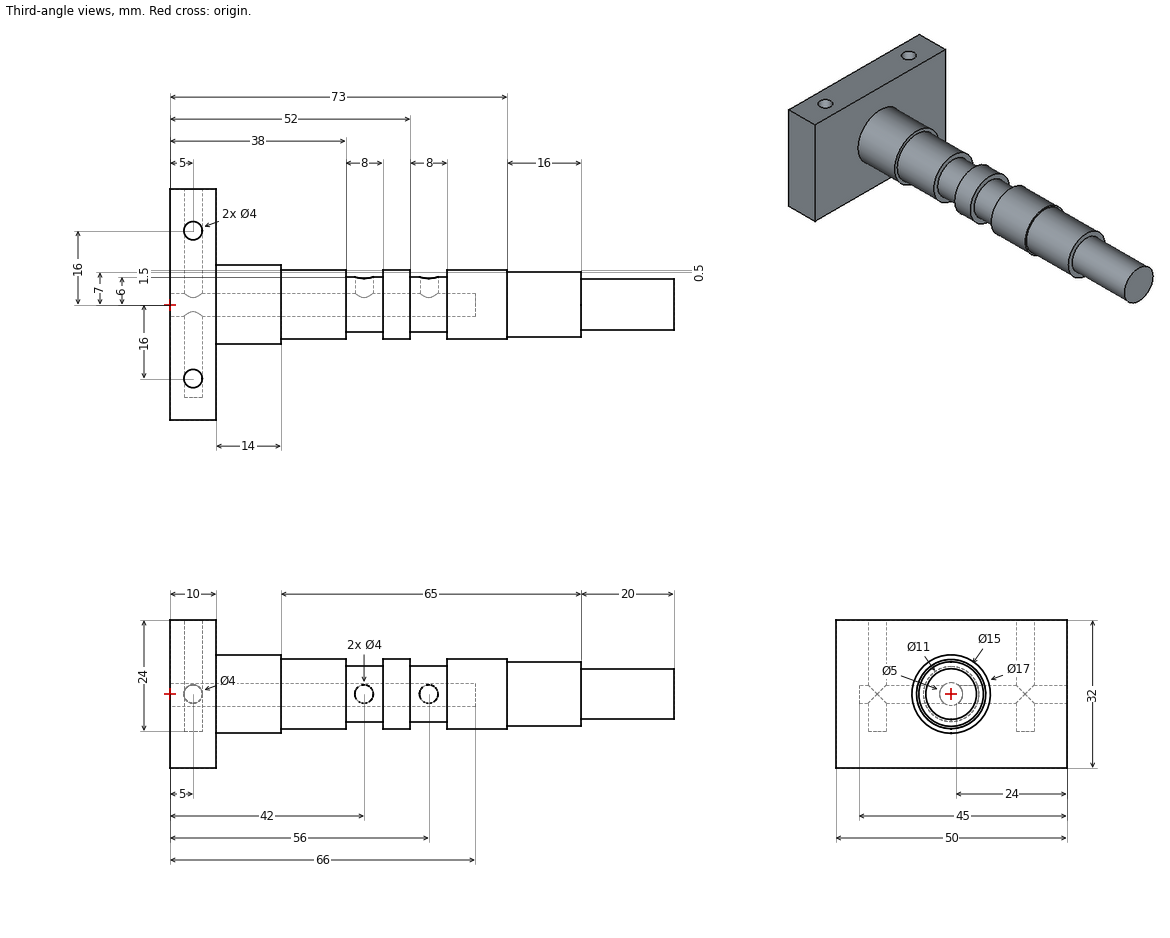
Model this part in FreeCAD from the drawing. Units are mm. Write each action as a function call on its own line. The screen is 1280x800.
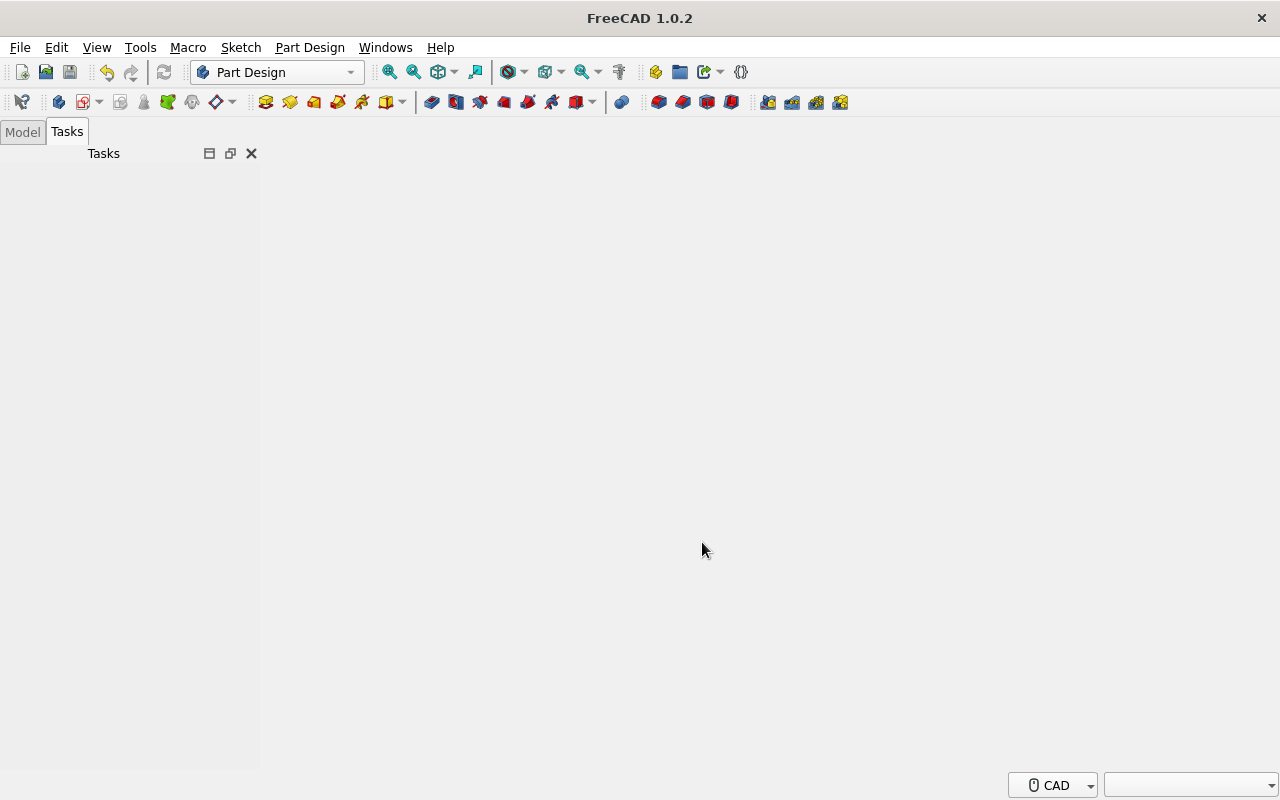
click(22, 72)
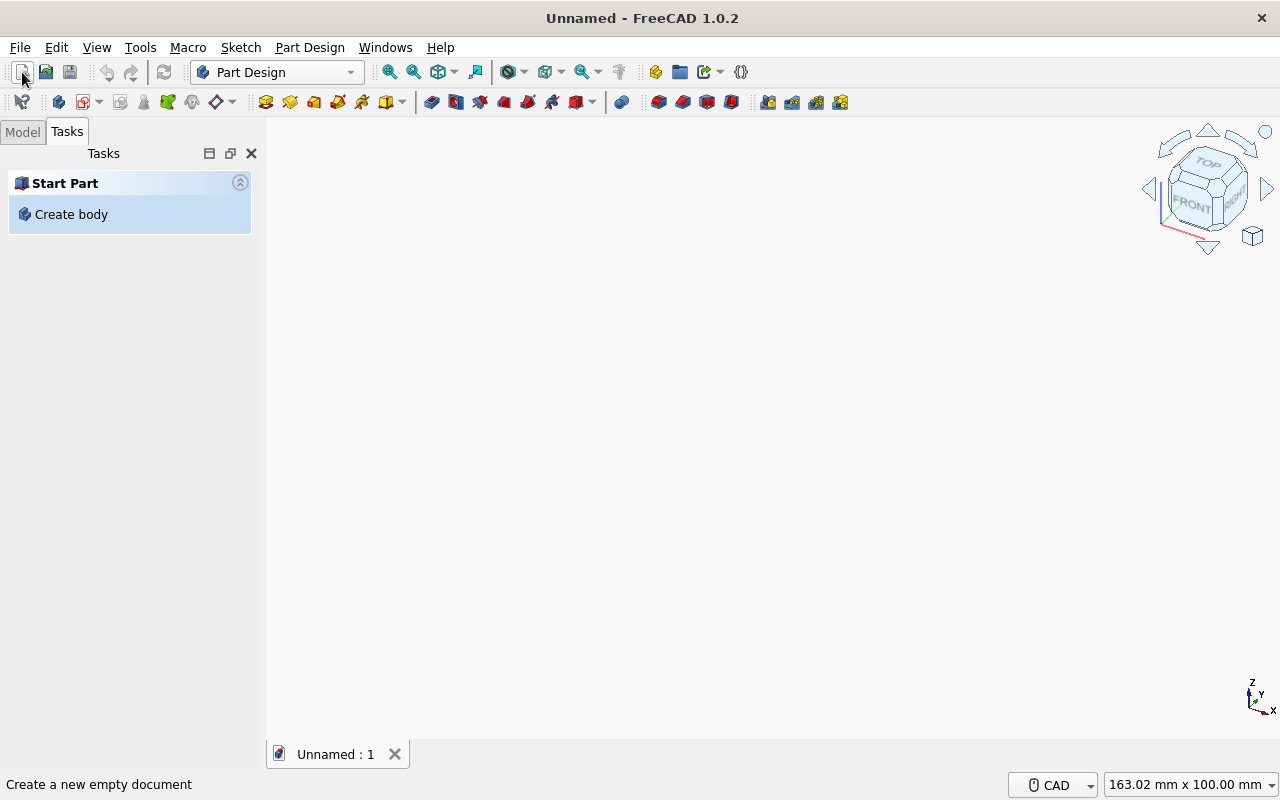
click(84, 102)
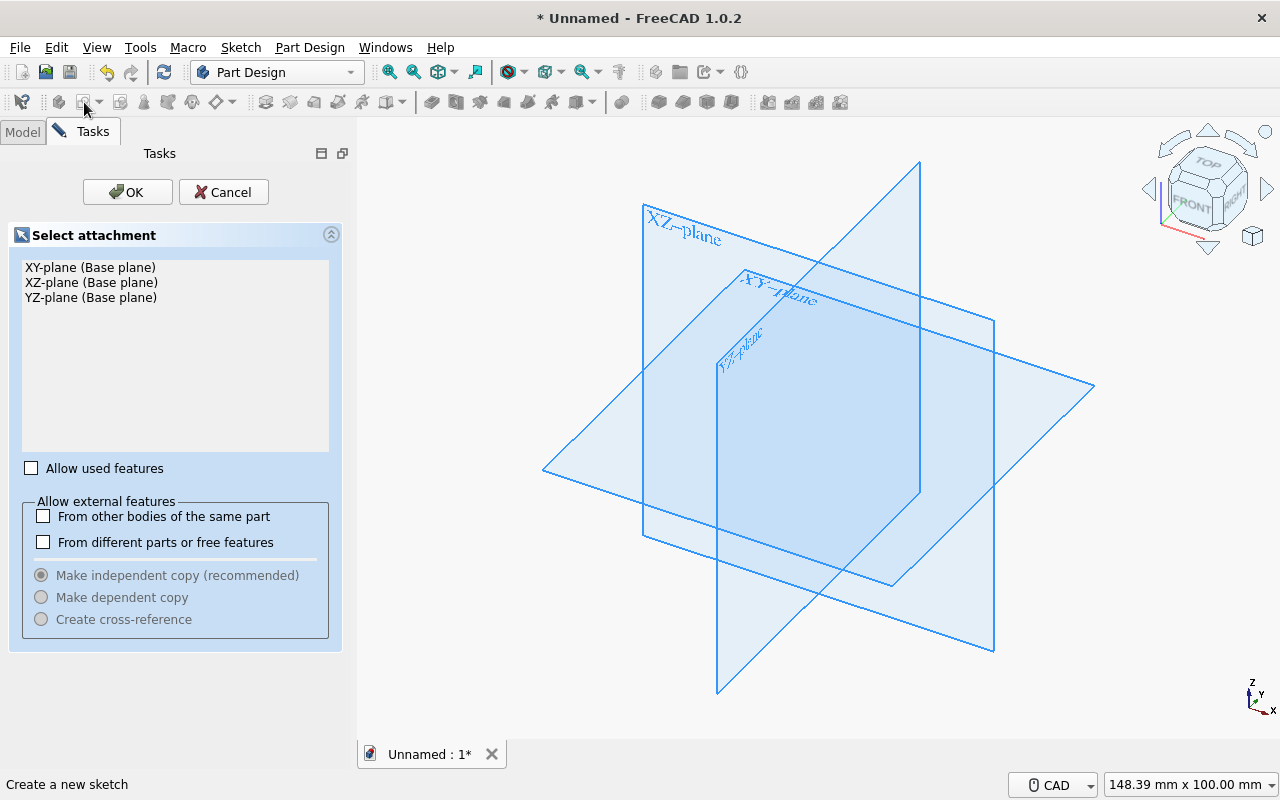
click(82, 298)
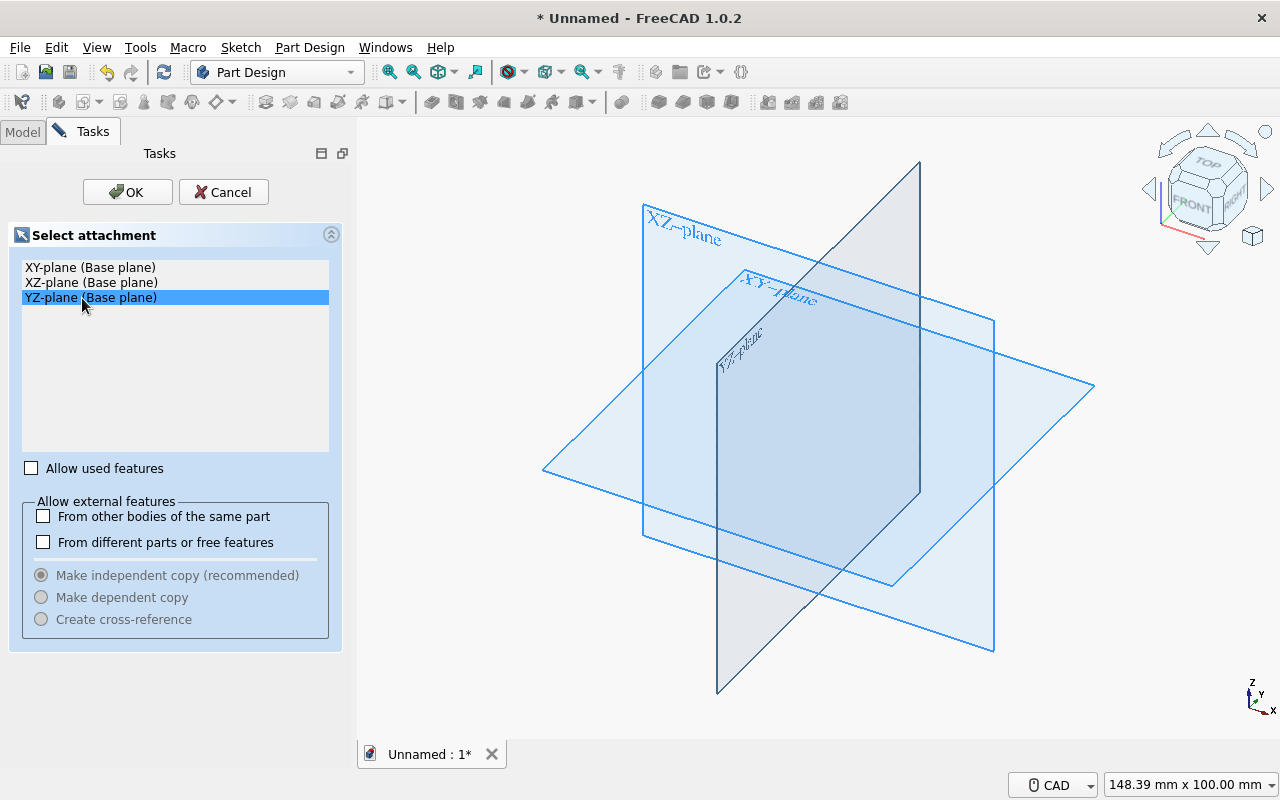
click(128, 192)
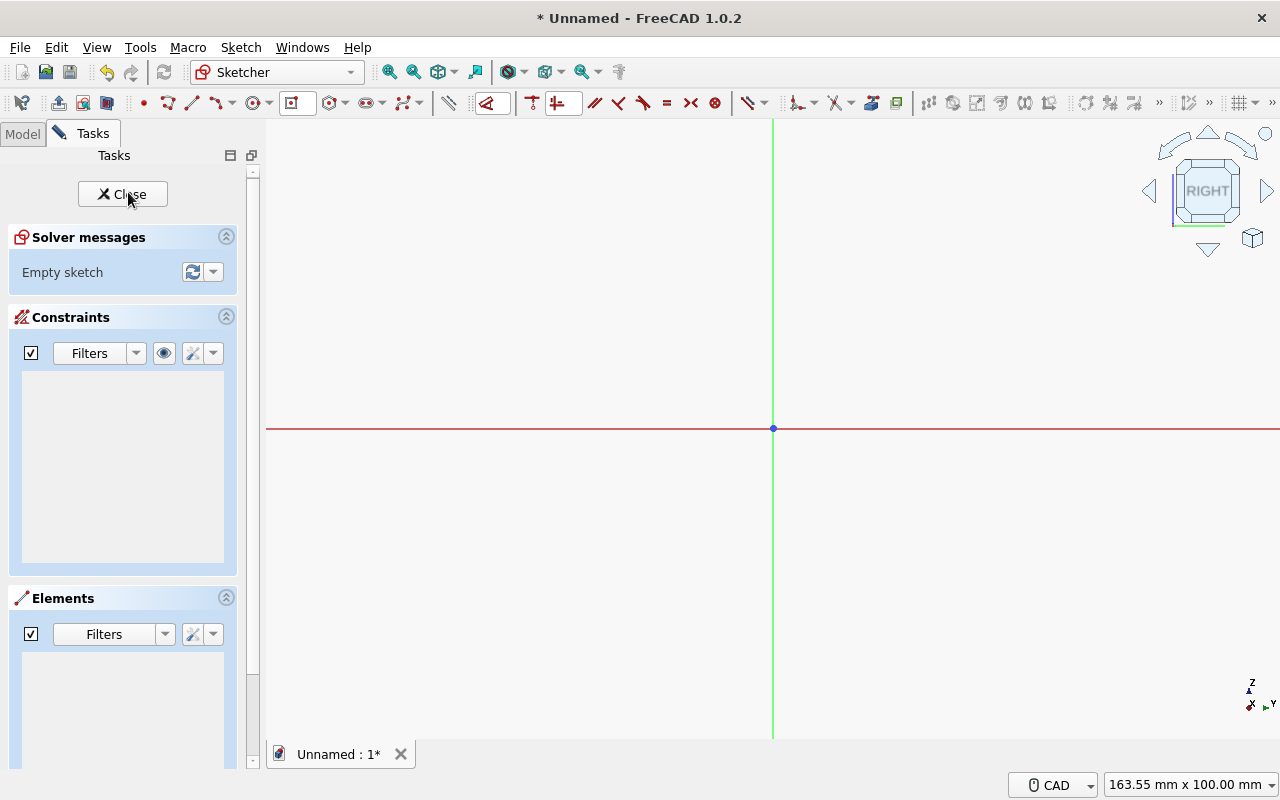
scroll(856, 429, up, 3)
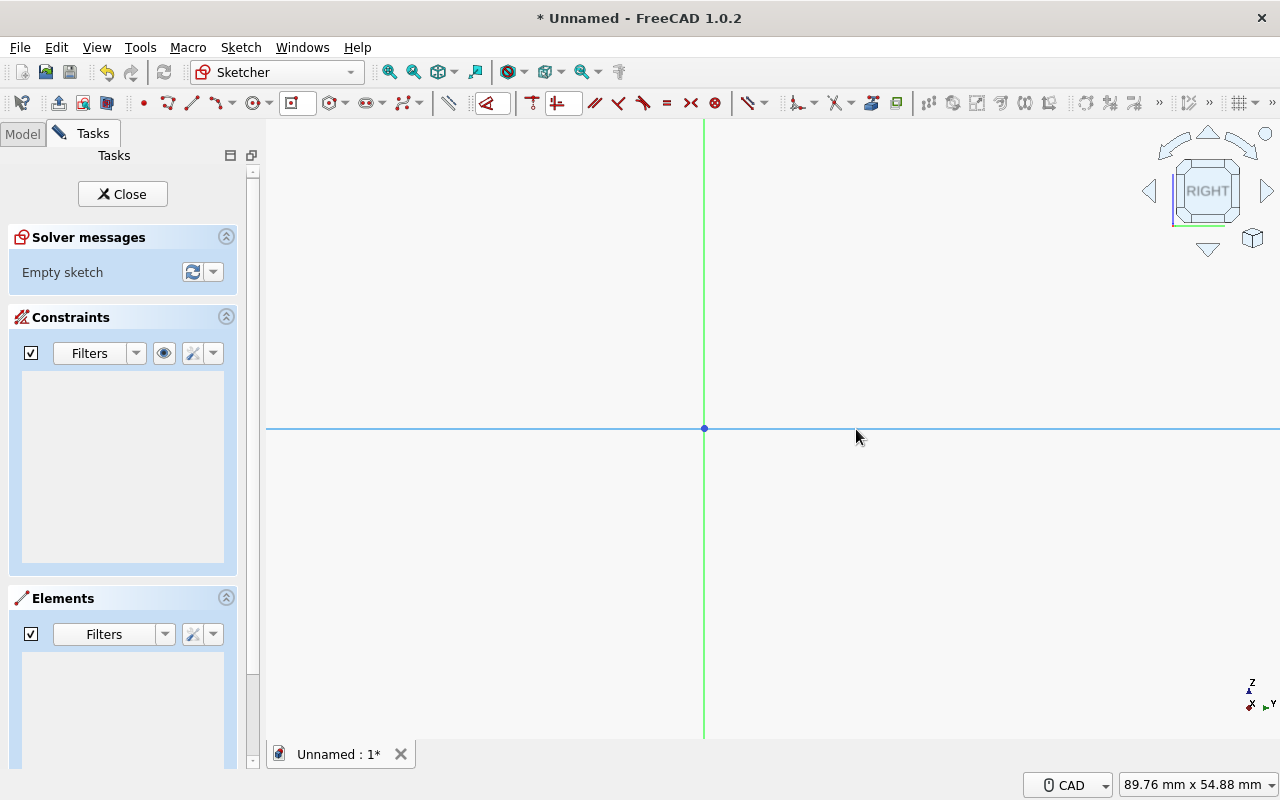
click(292, 104)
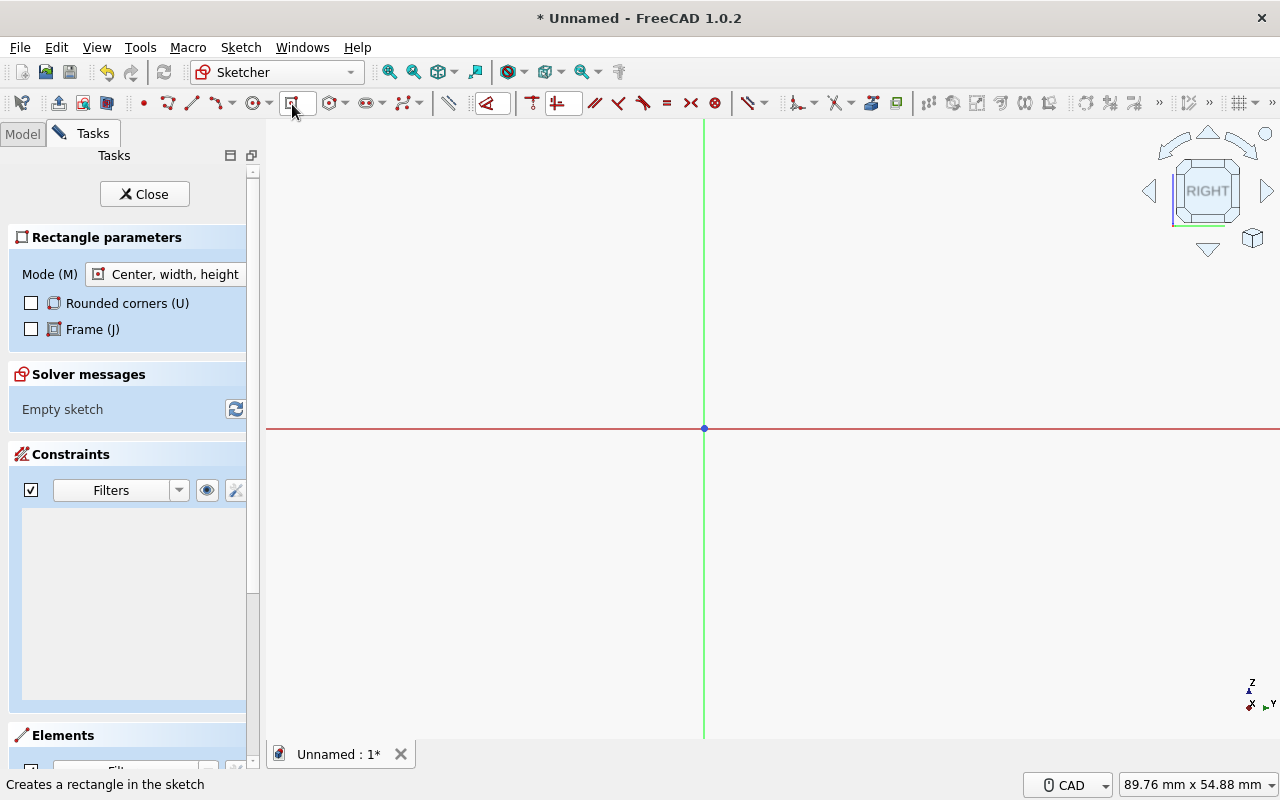
click(704, 429)
move(987, 248)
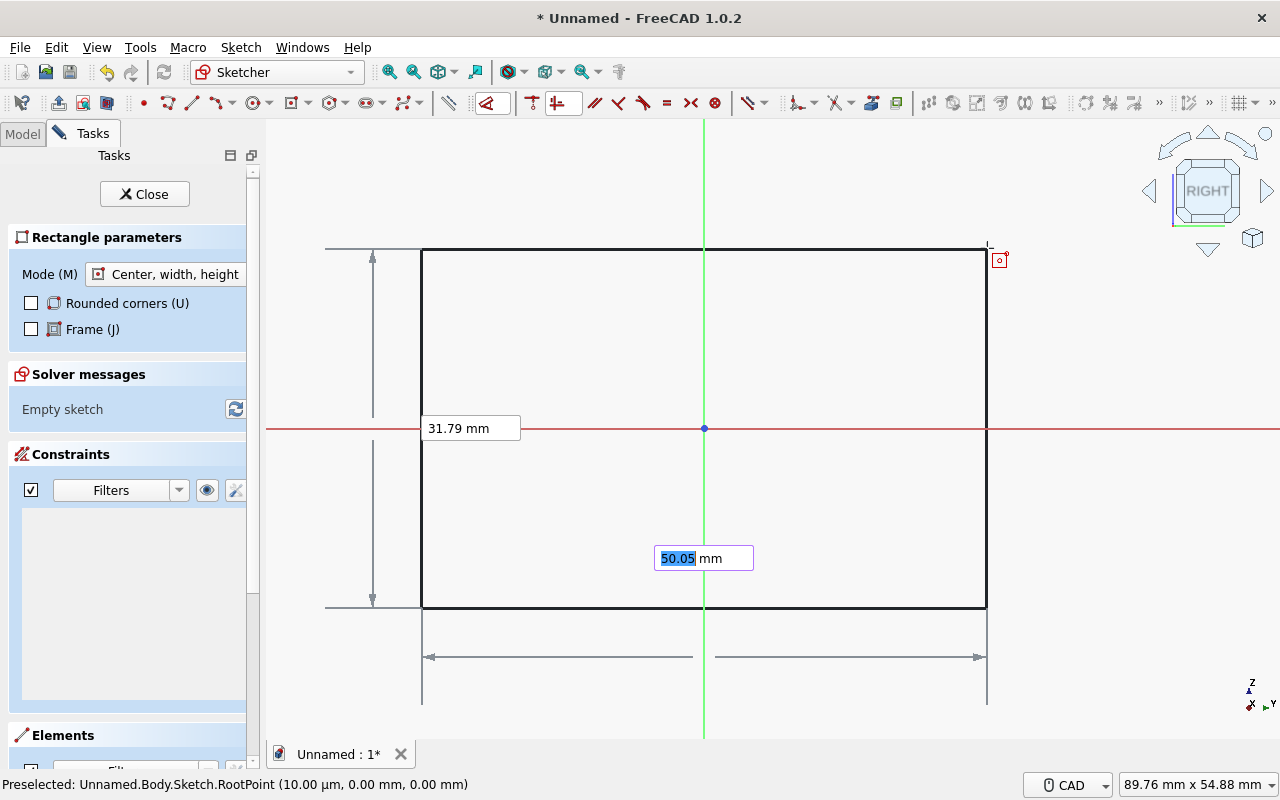
text(50)
key(Tab)
text(32)
key(Return)
key(Escape)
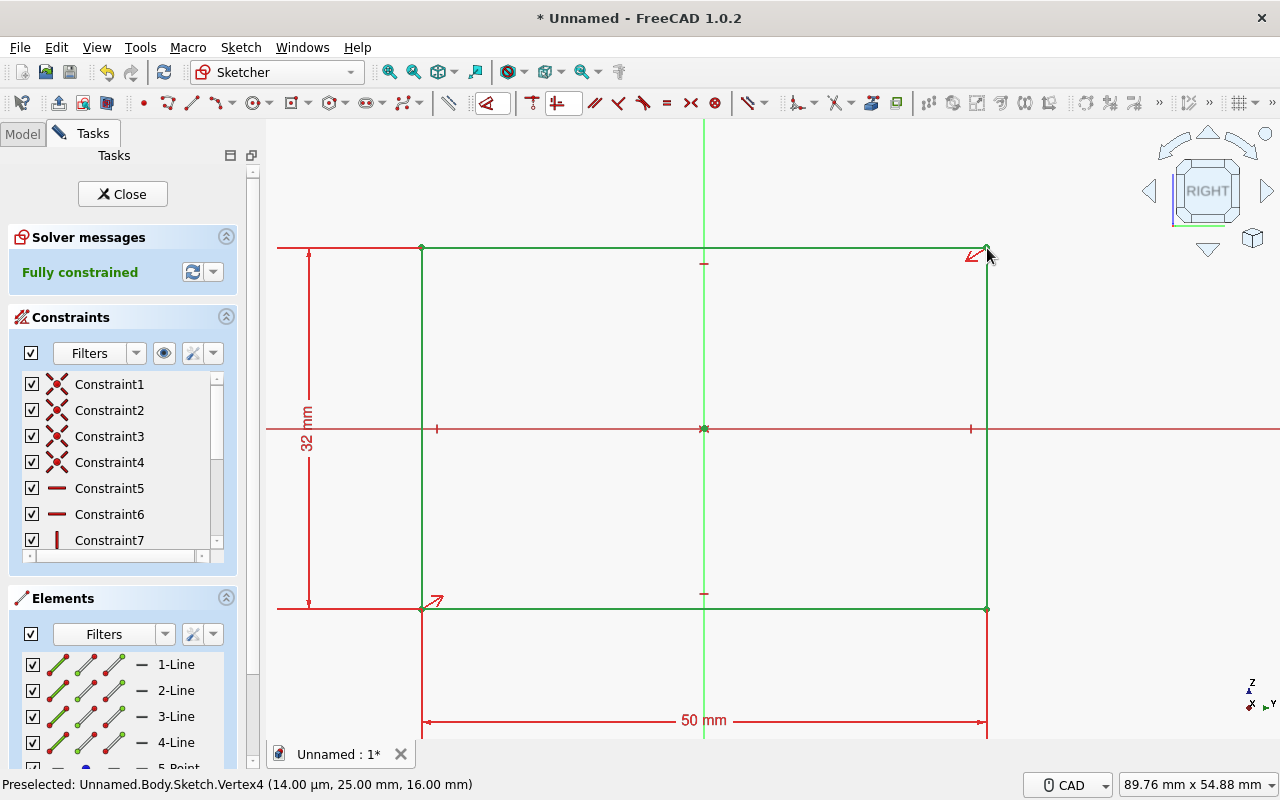
click(123, 194)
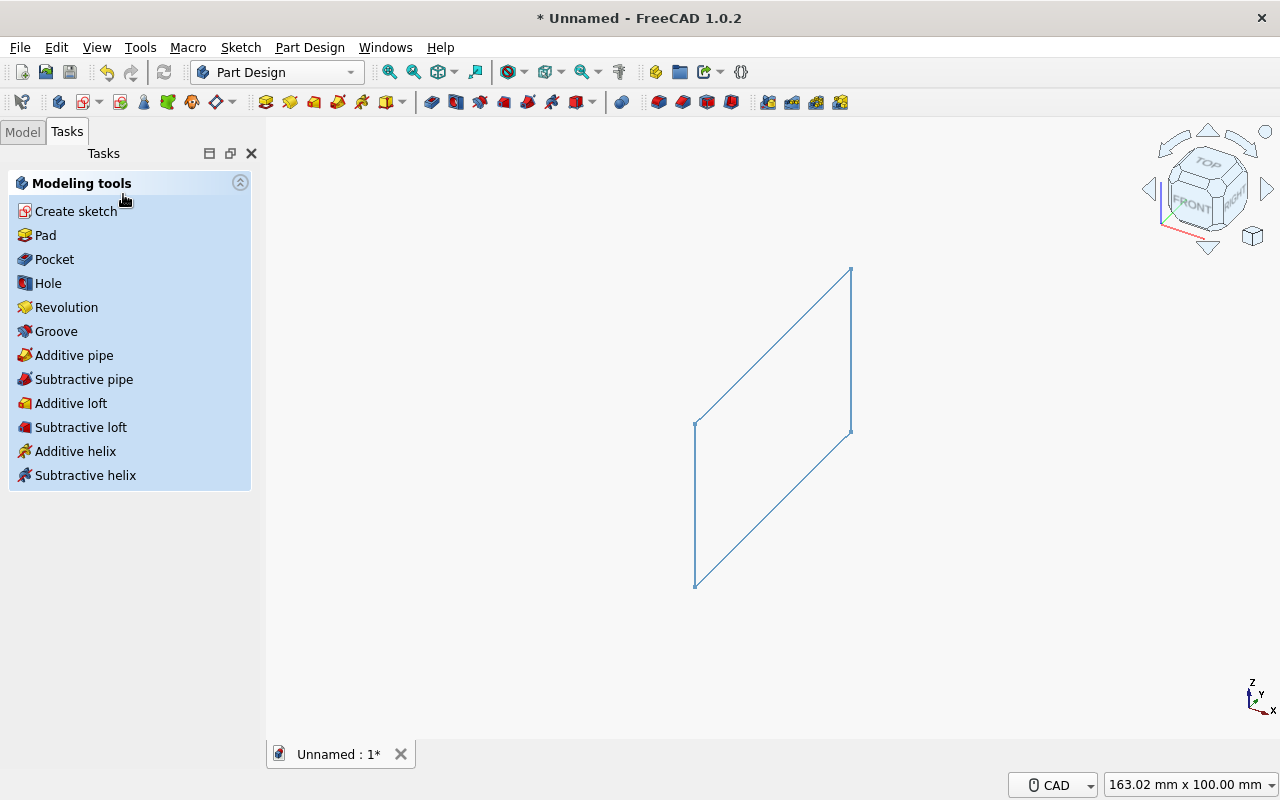
click(266, 102)